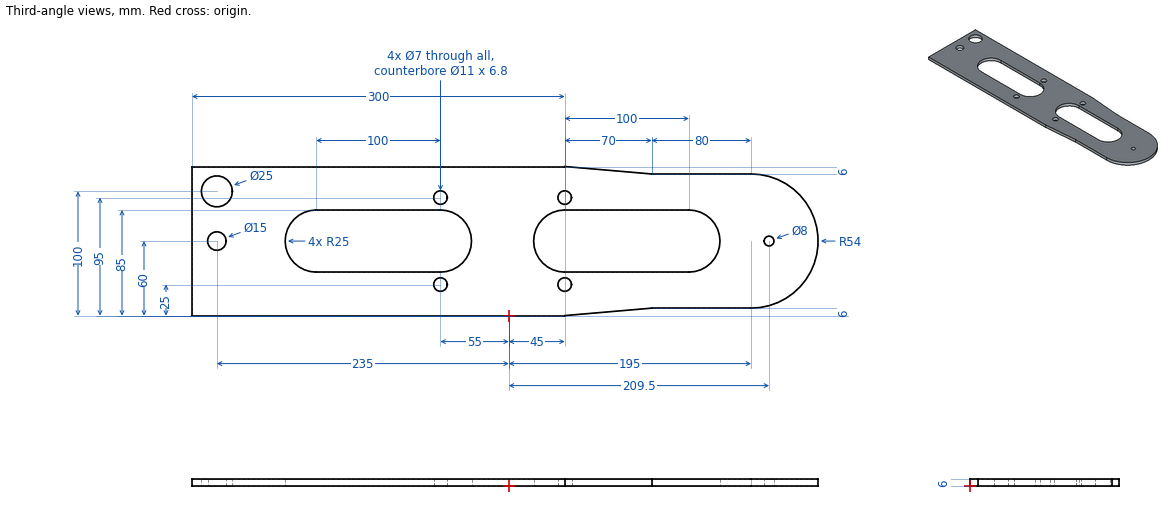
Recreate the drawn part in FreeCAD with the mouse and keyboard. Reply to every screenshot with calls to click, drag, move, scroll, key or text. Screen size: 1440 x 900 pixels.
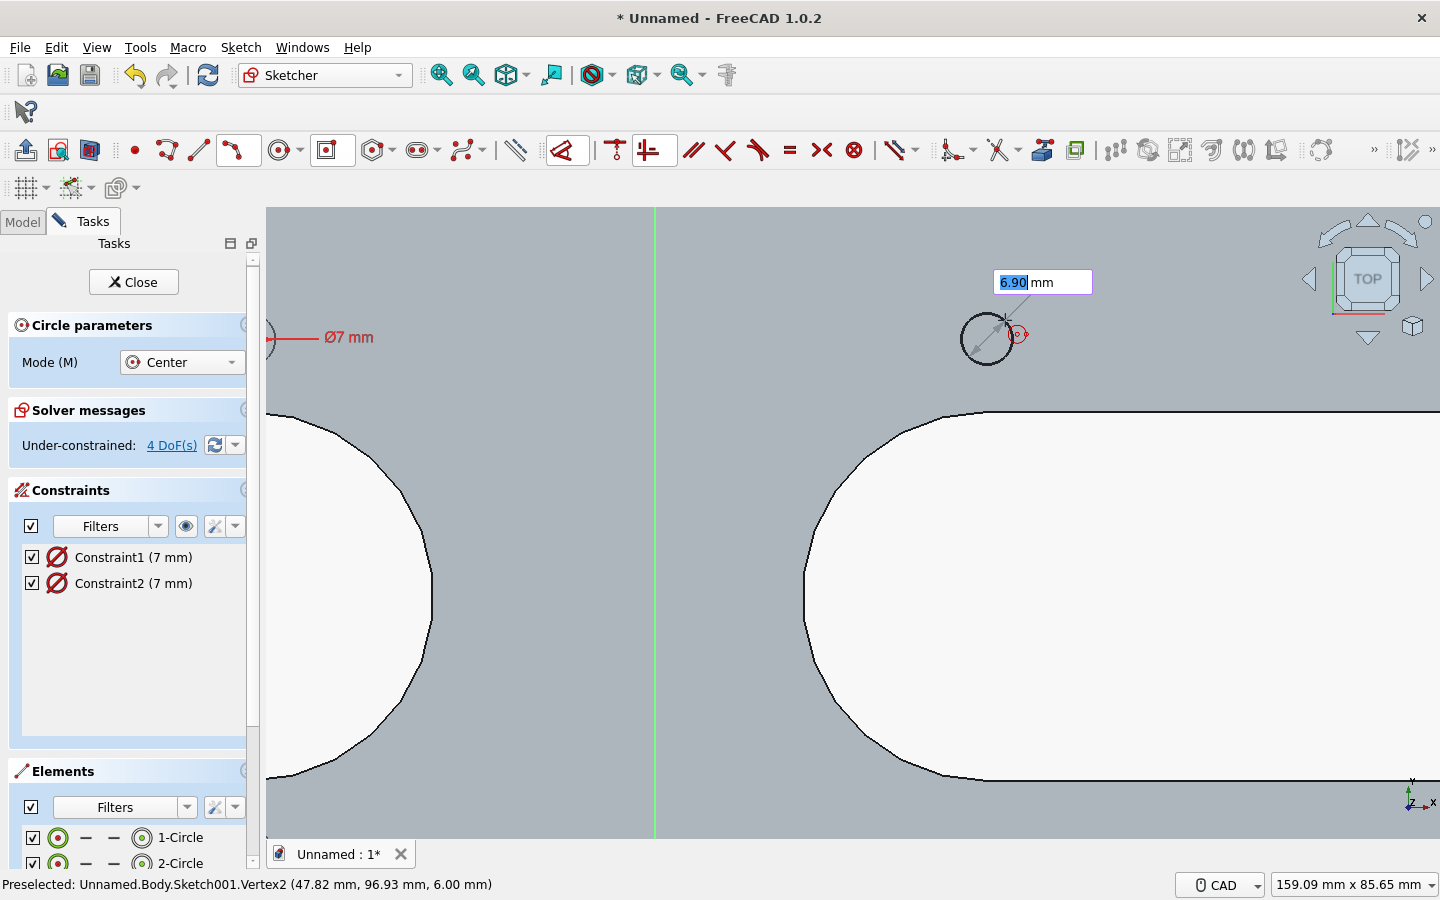
text(7)
key(Return)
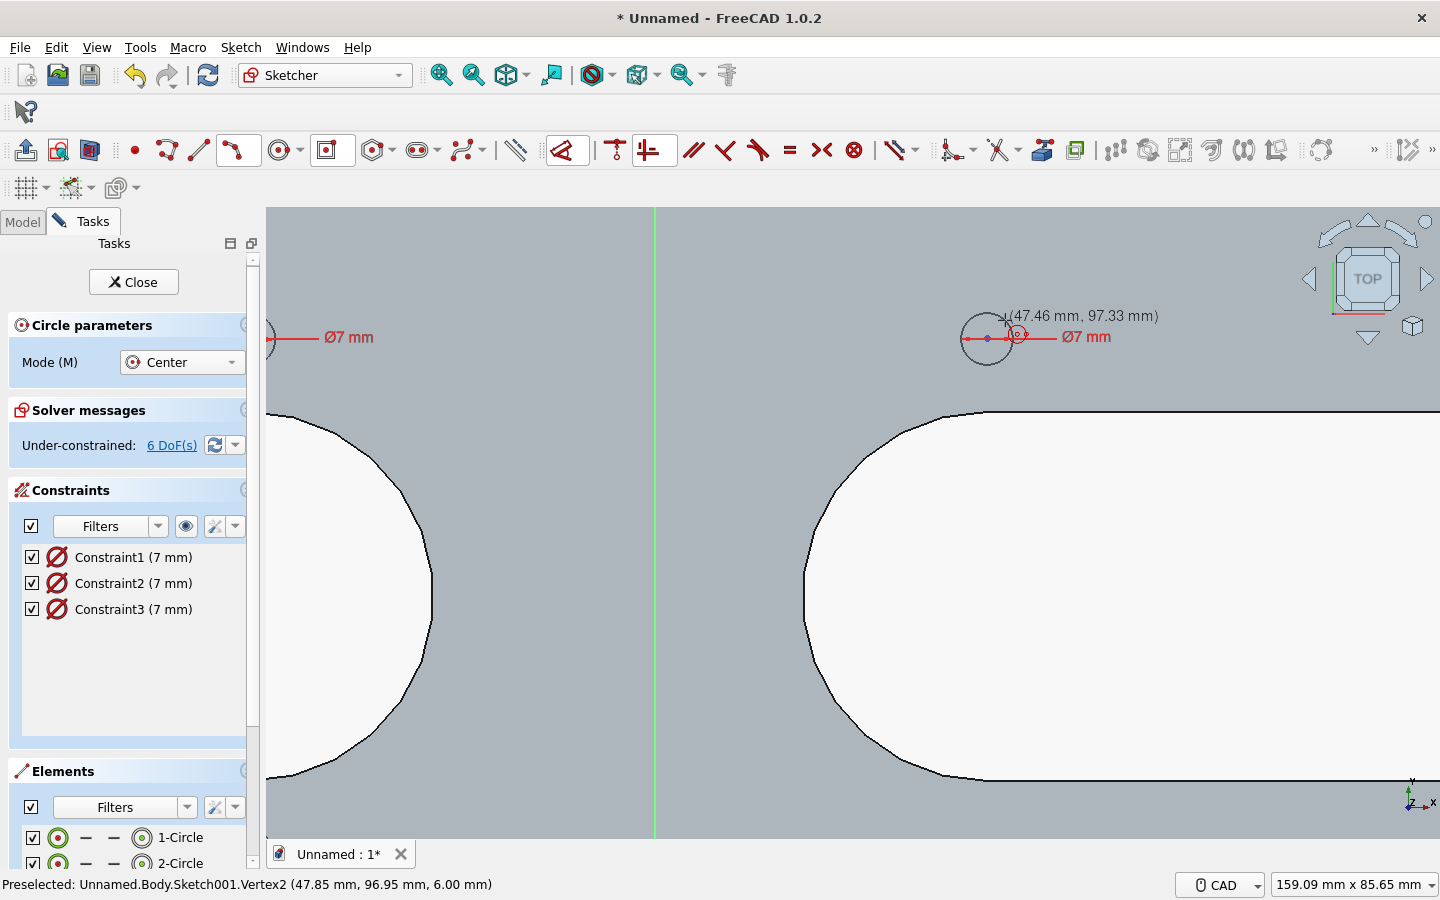
scroll(987, 337, down, 3)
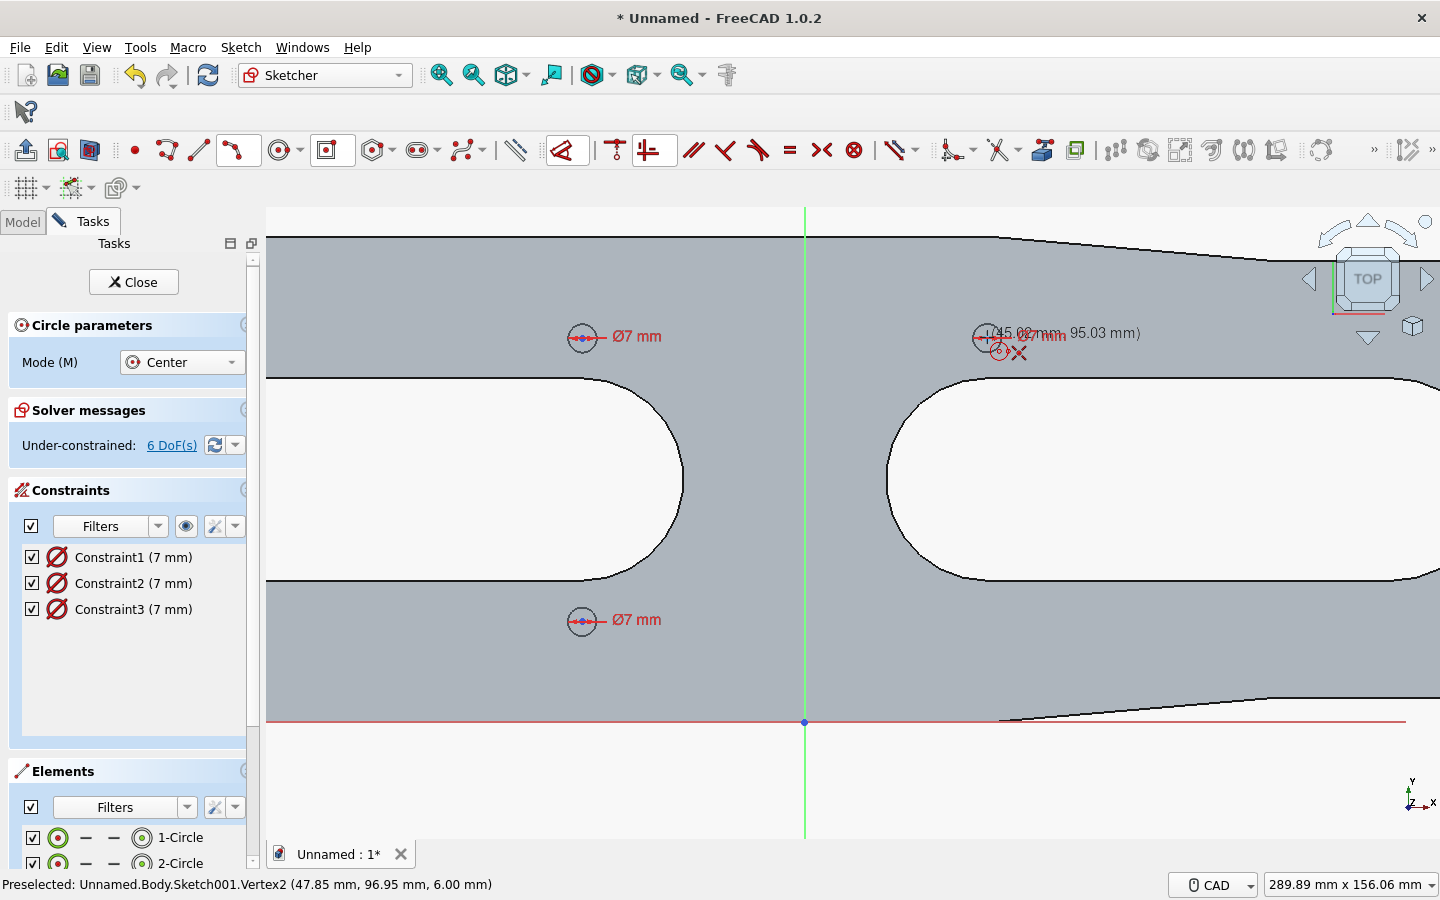
scroll(987, 621, up, 3)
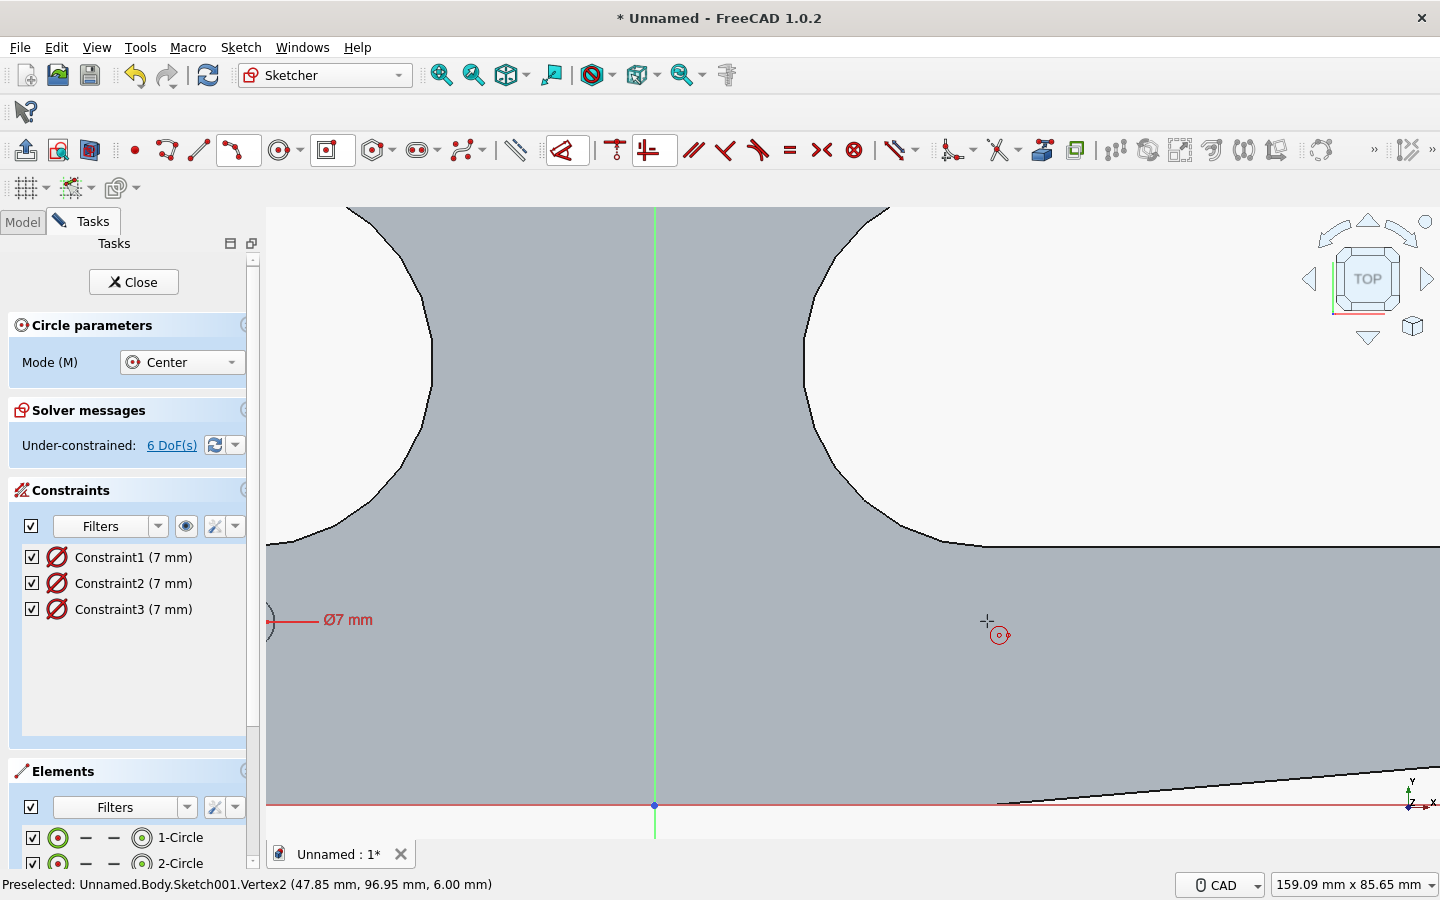
click(987, 621)
move(1005, 603)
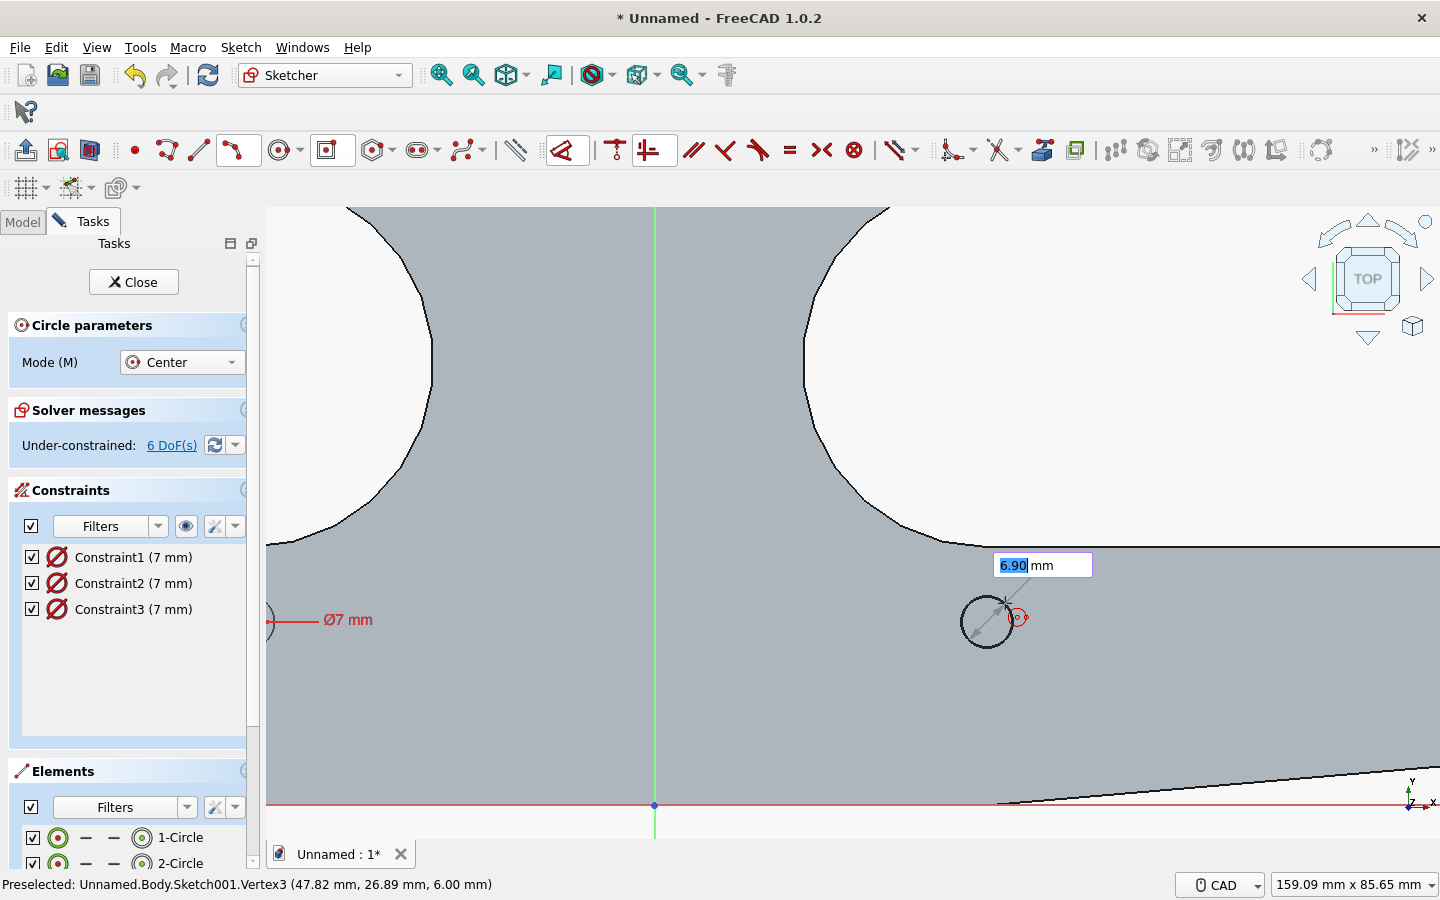
text(7)
key(Return)
key(Escape)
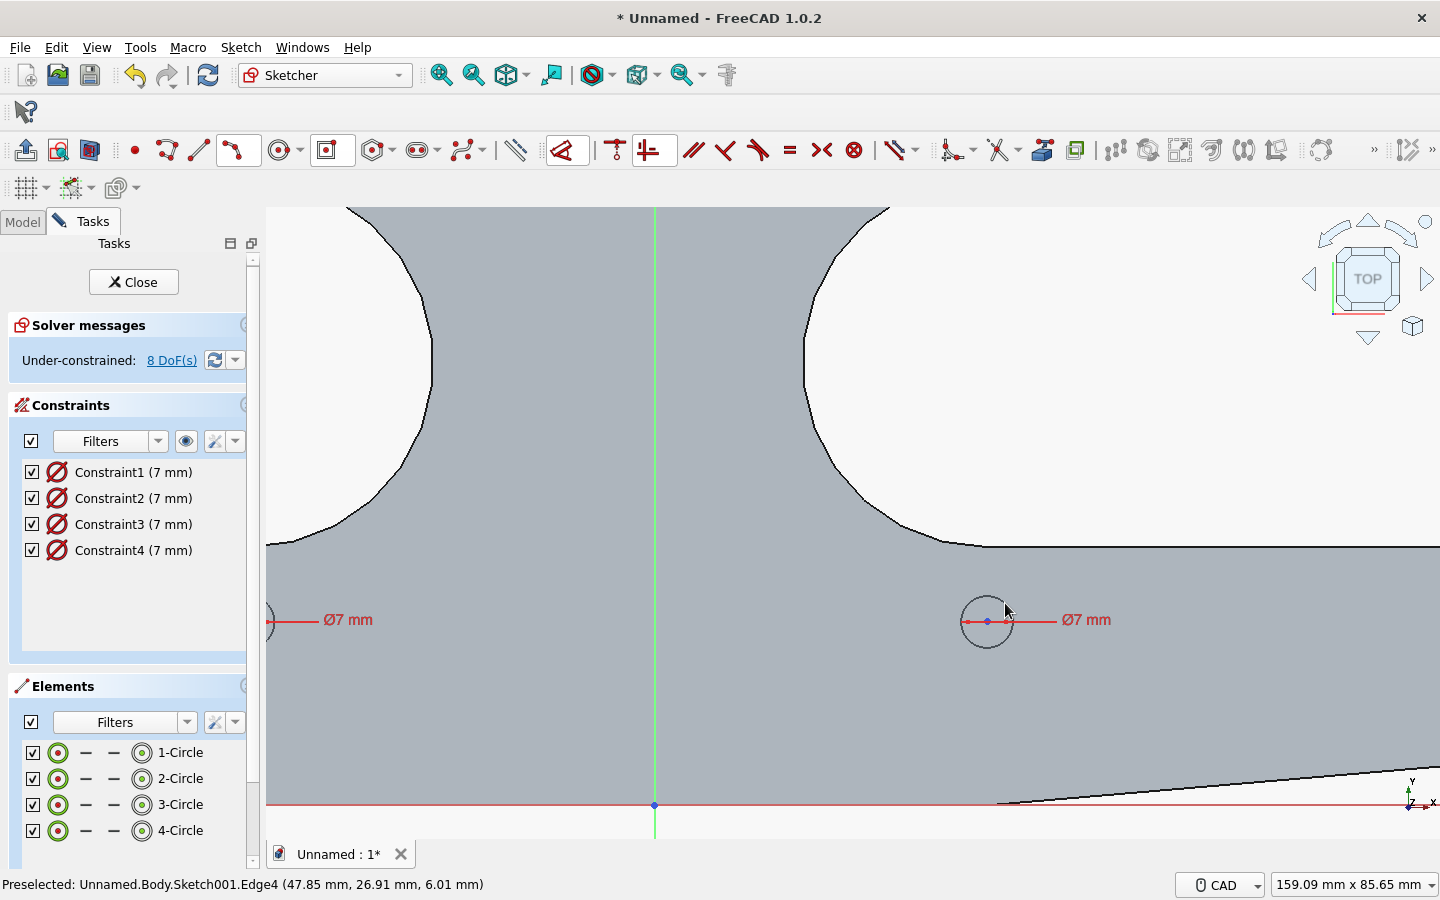
scroll(987, 622, down, 3)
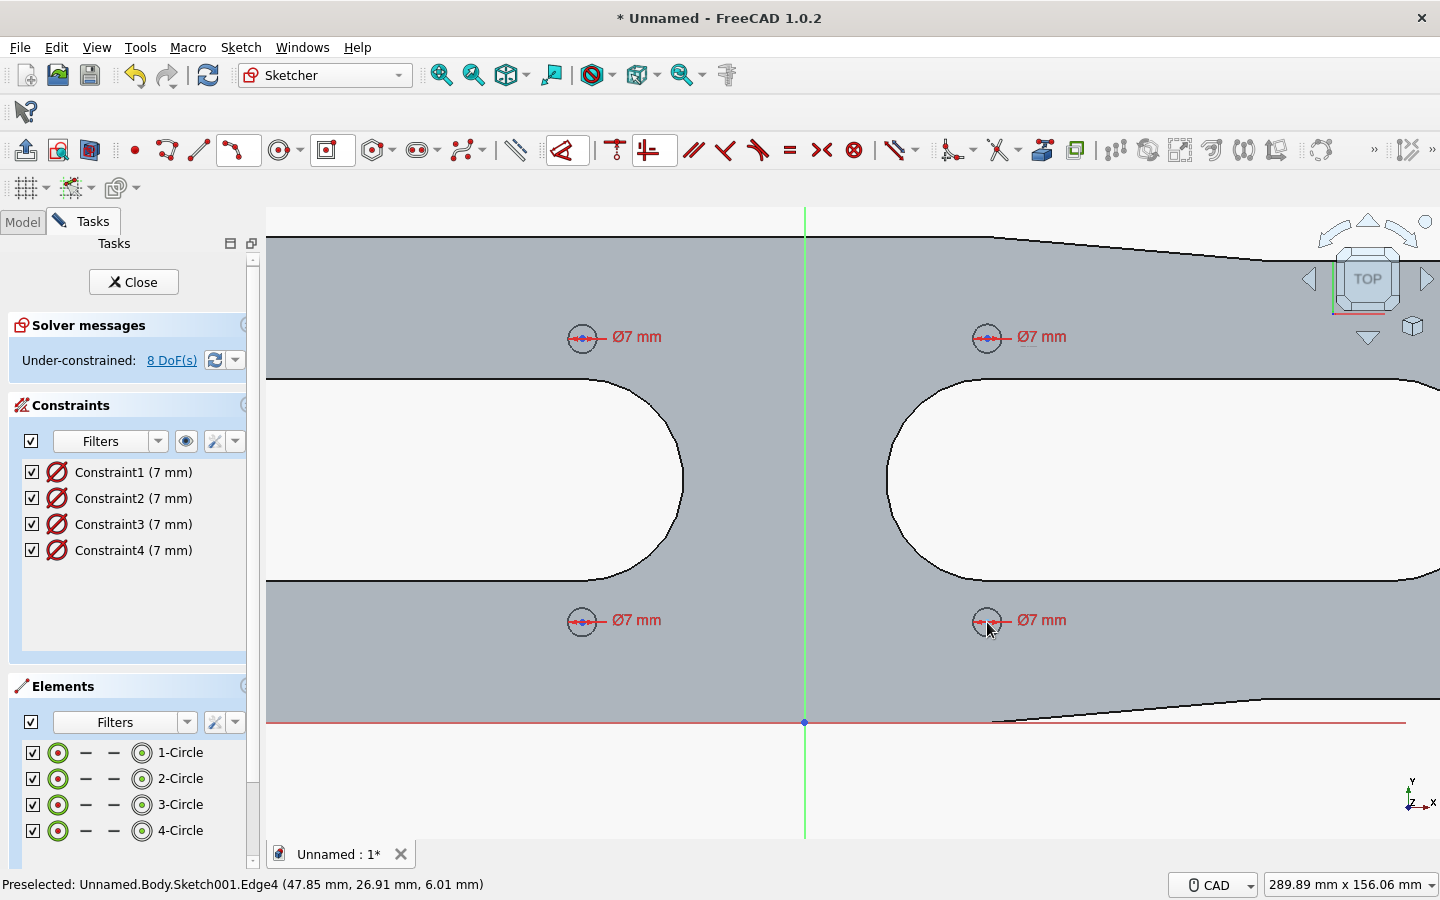
click(582, 339)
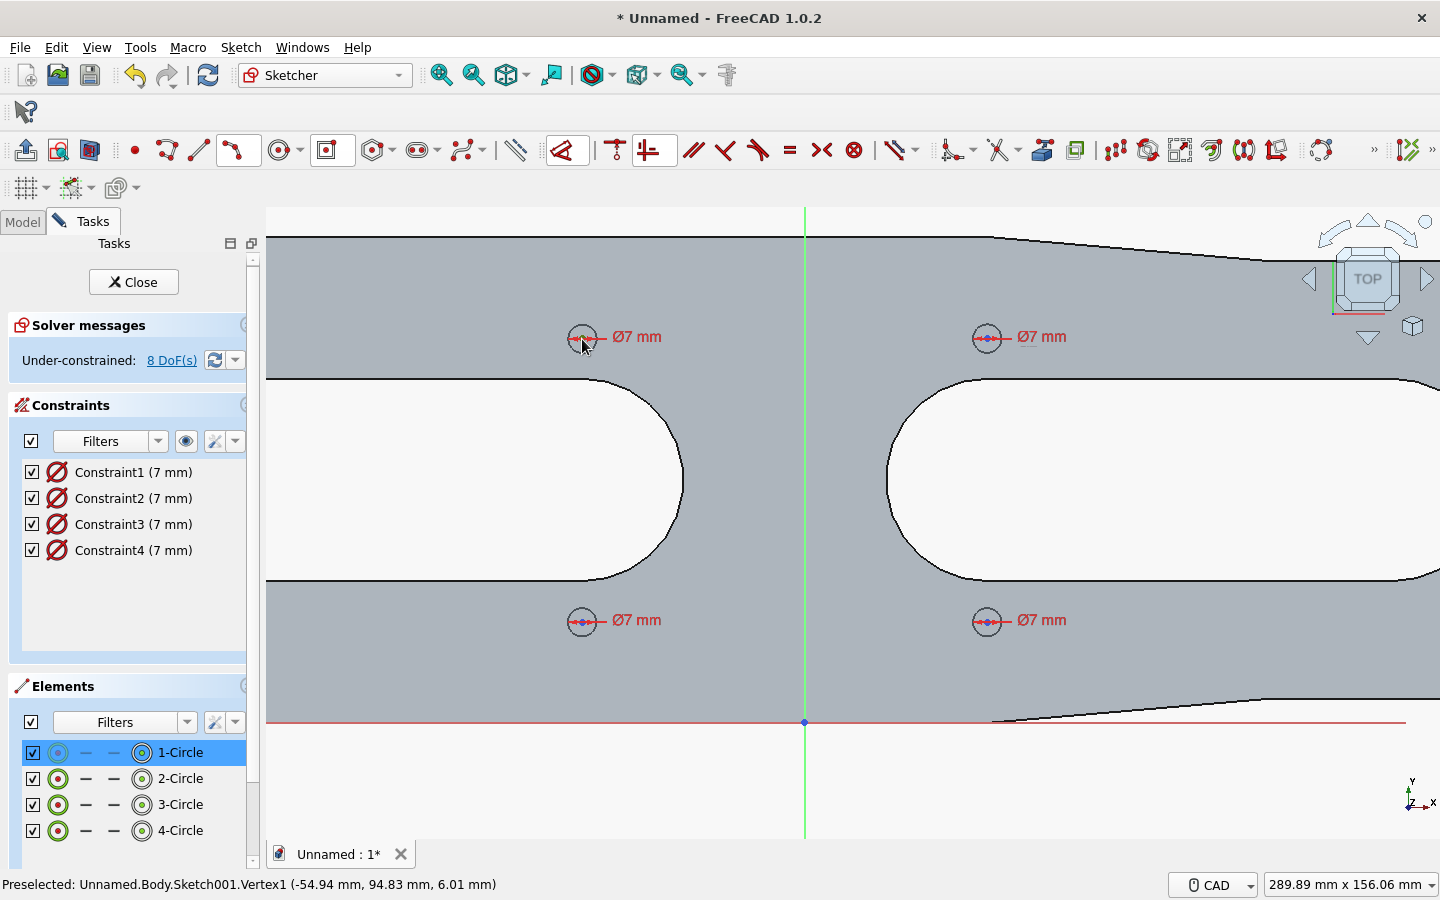
click(582, 622)